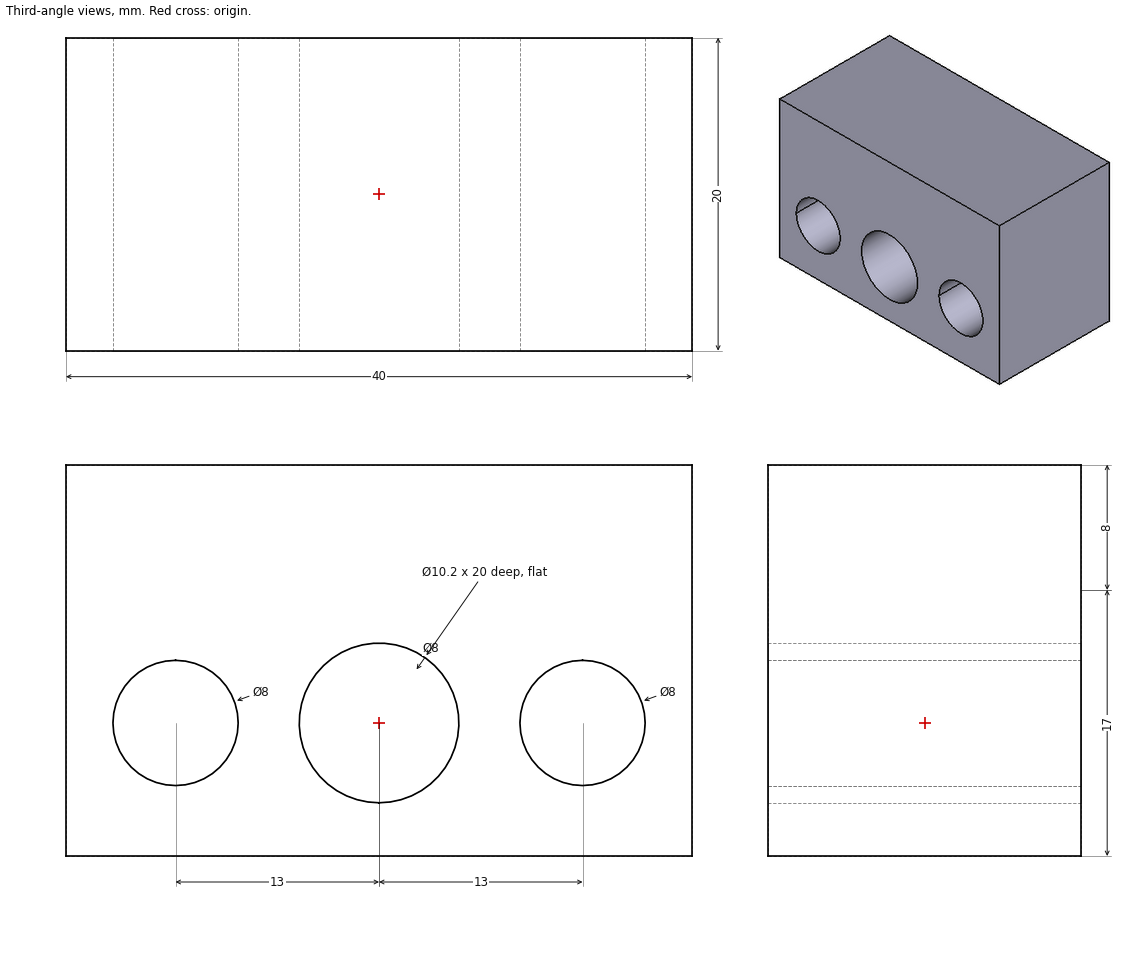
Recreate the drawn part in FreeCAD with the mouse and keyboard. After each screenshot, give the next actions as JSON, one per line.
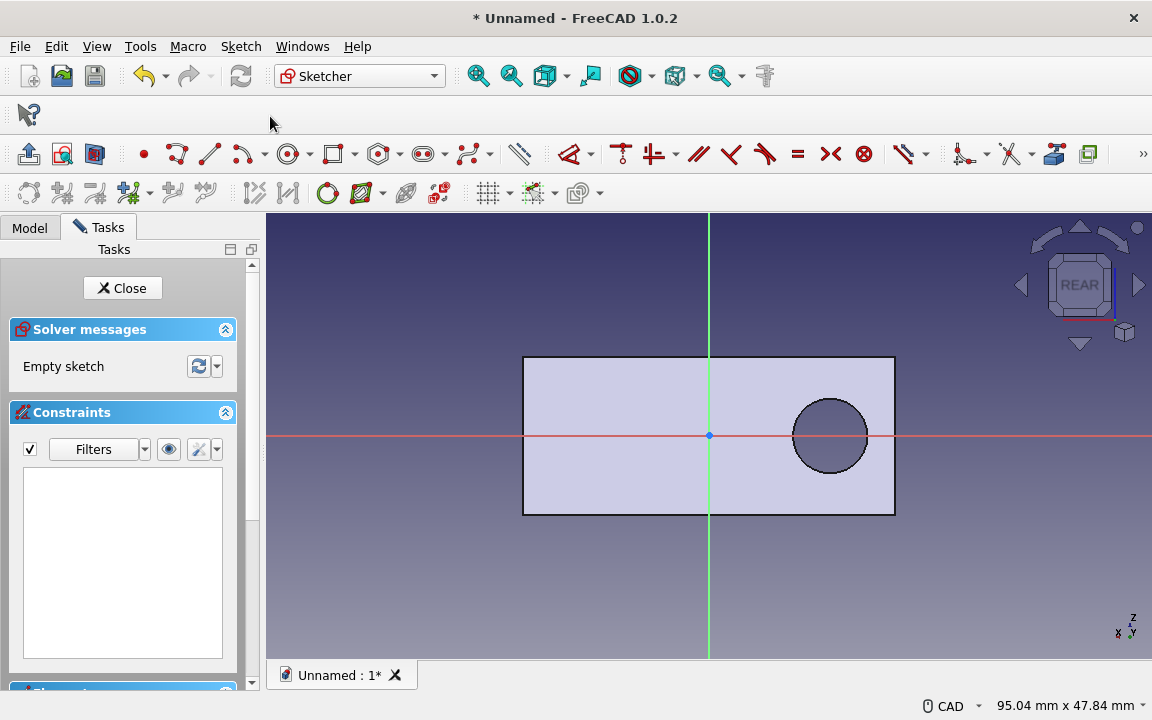
{"action": "scroll", "coordinate": [625, 436], "scroll_direction": "up", "scroll_amount": 6}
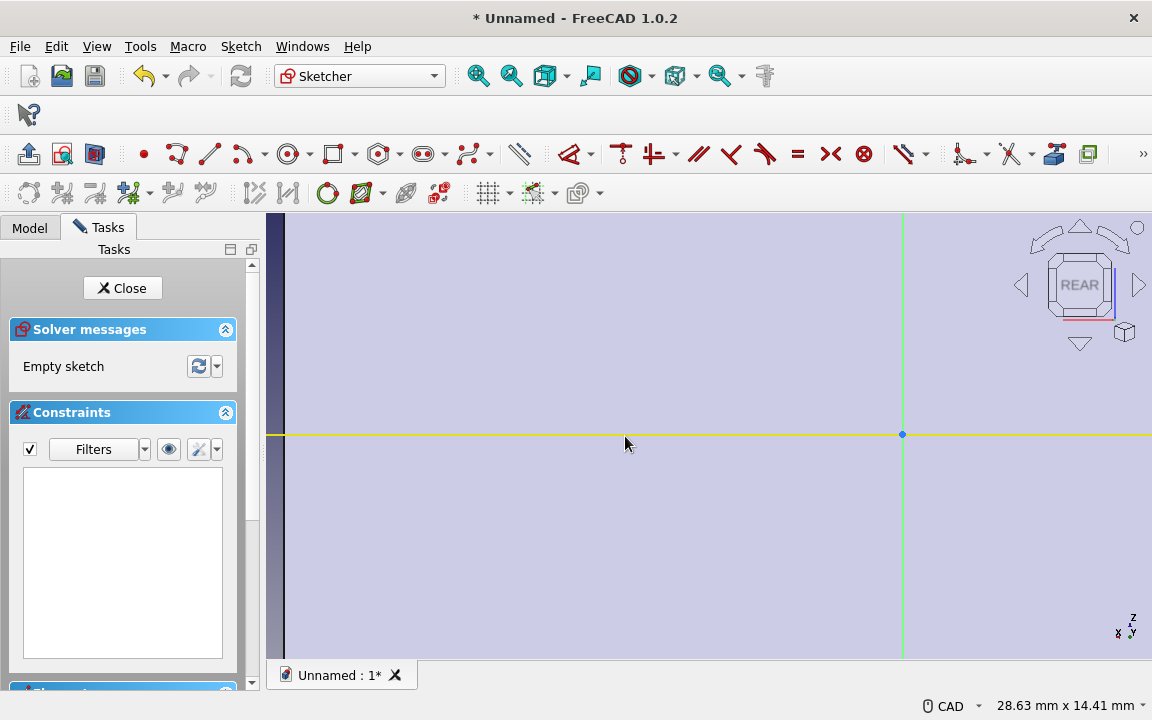
{"action": "left_click", "coordinate": [288, 154]}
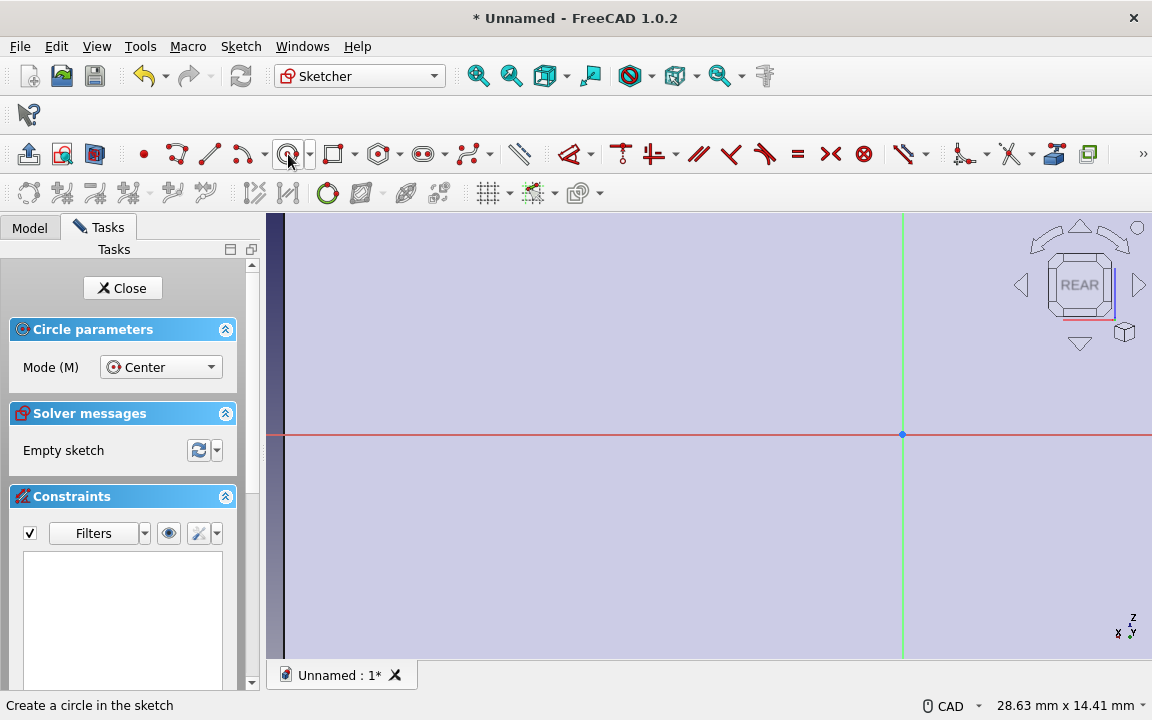
{"action": "left_click", "coordinate": [501, 435]}
{"action": "left_click", "coordinate": [588, 347]}
{"action": "key", "text": "Escape"}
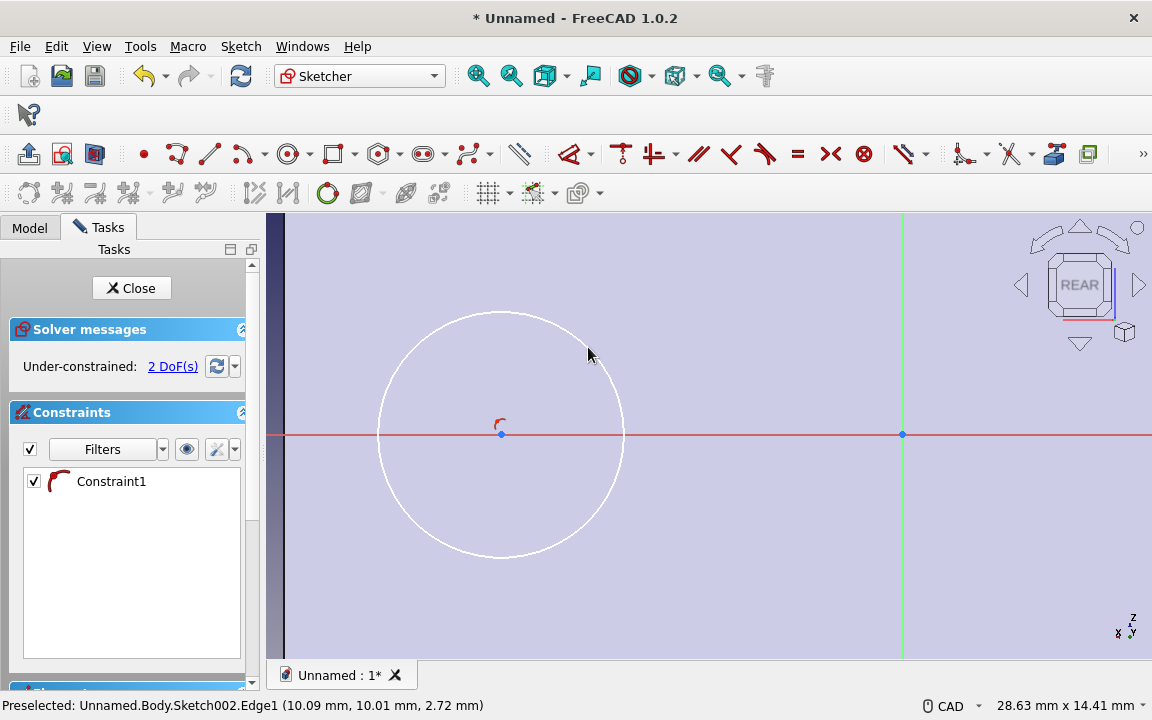
{"action": "left_click", "coordinate": [568, 154]}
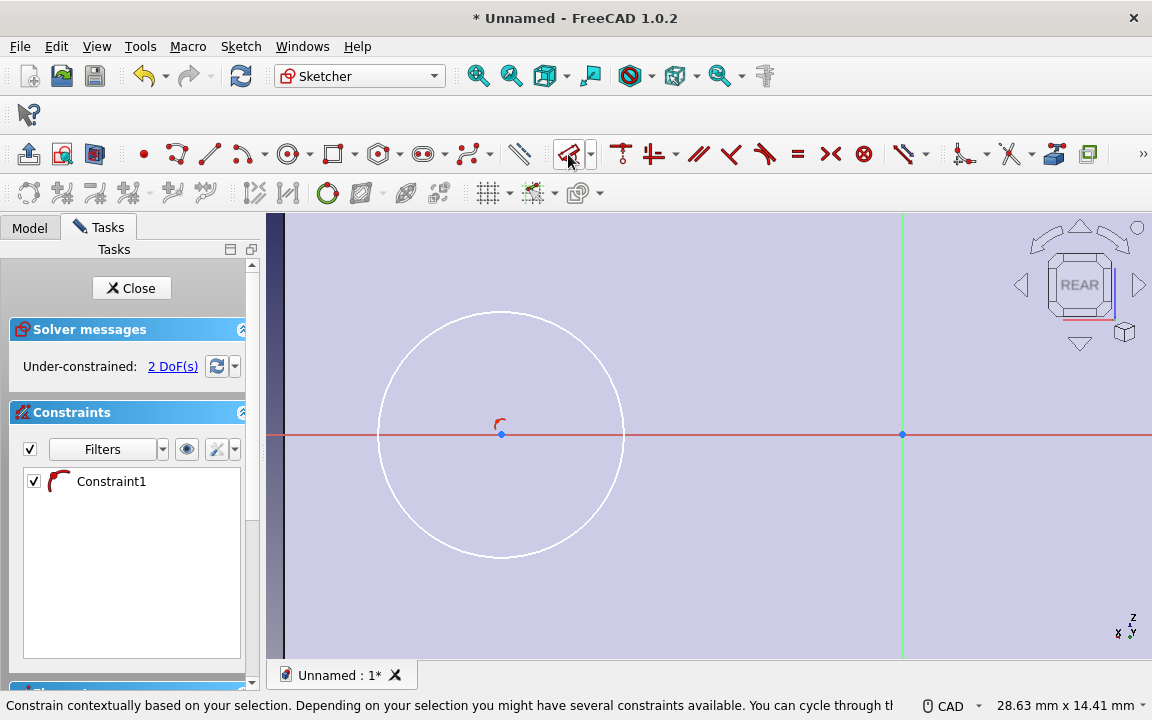
{"action": "left_click", "coordinate": [588, 348]}
{"action": "left_click", "coordinate": [611, 325]}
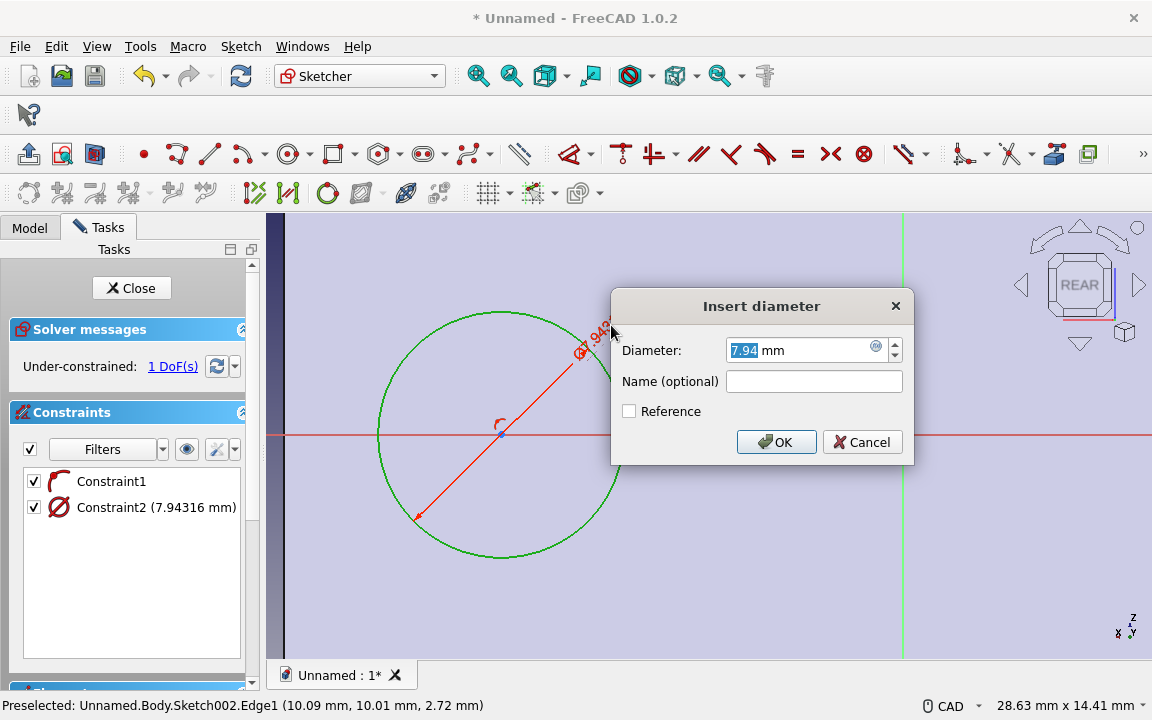
{"action": "type", "text": "8"}
{"action": "key", "text": "Return"}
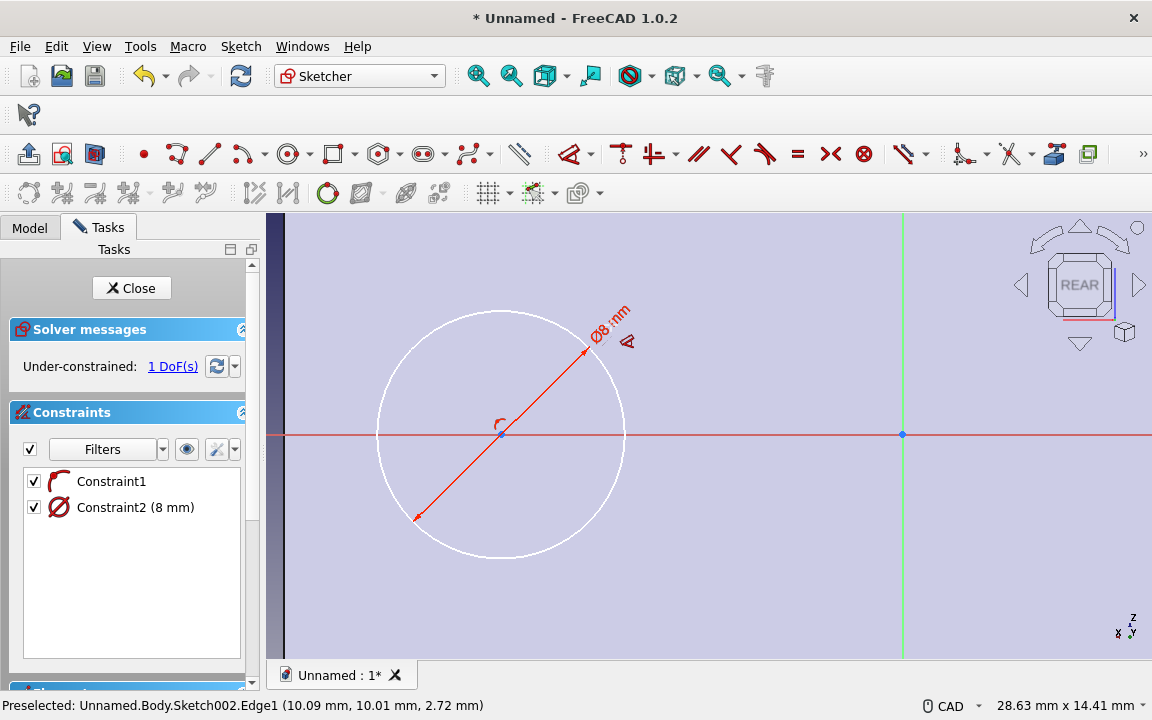
{"action": "left_click", "coordinate": [501, 435]}
{"action": "left_click", "coordinate": [702, 469]}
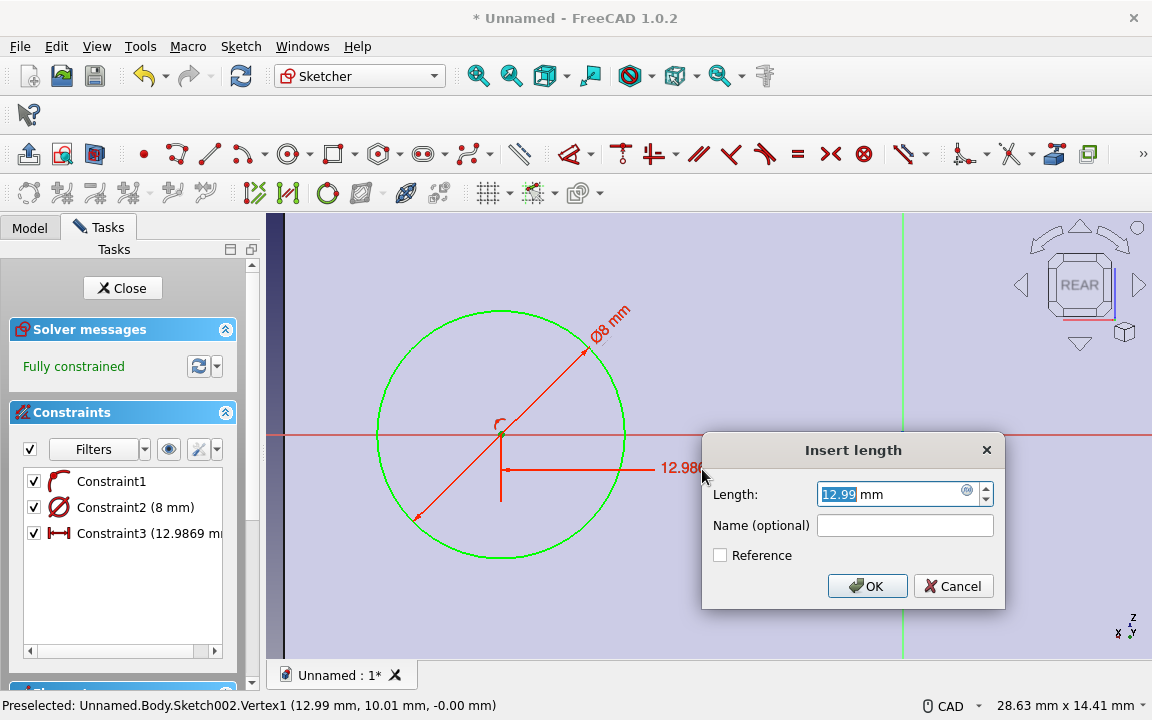
{"action": "type", "text": "13"}
{"action": "key", "text": "Return"}
{"action": "key", "text": "Escape"}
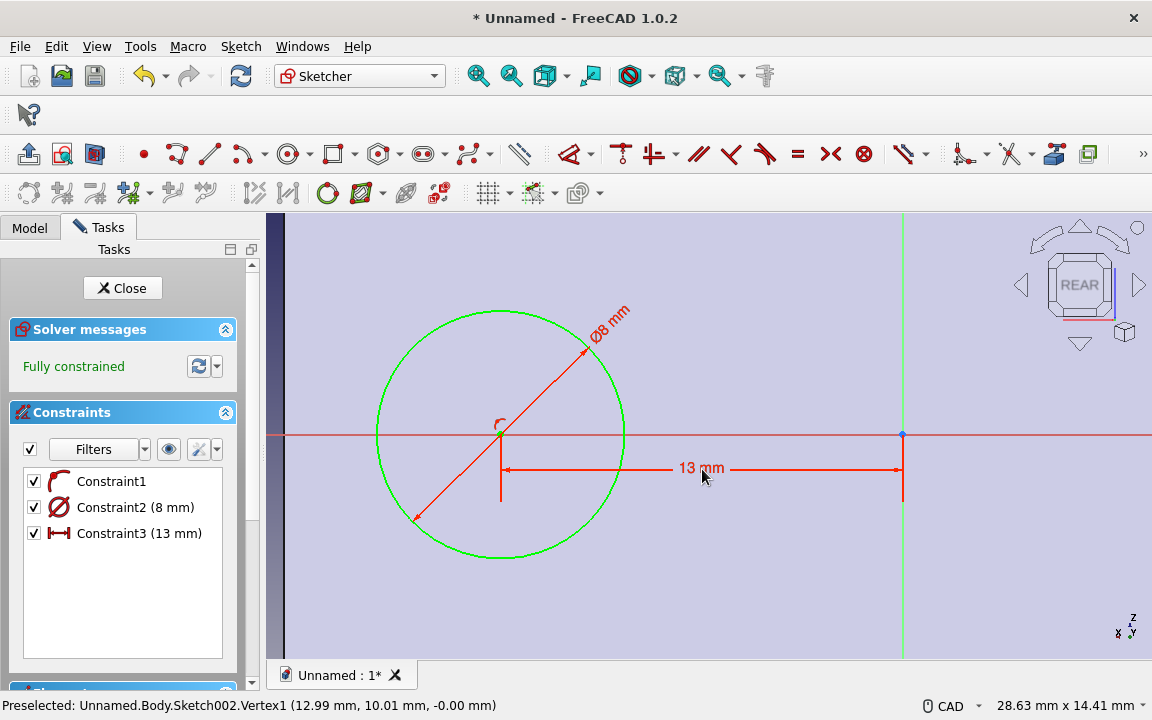
{"action": "left_click", "coordinate": [123, 288]}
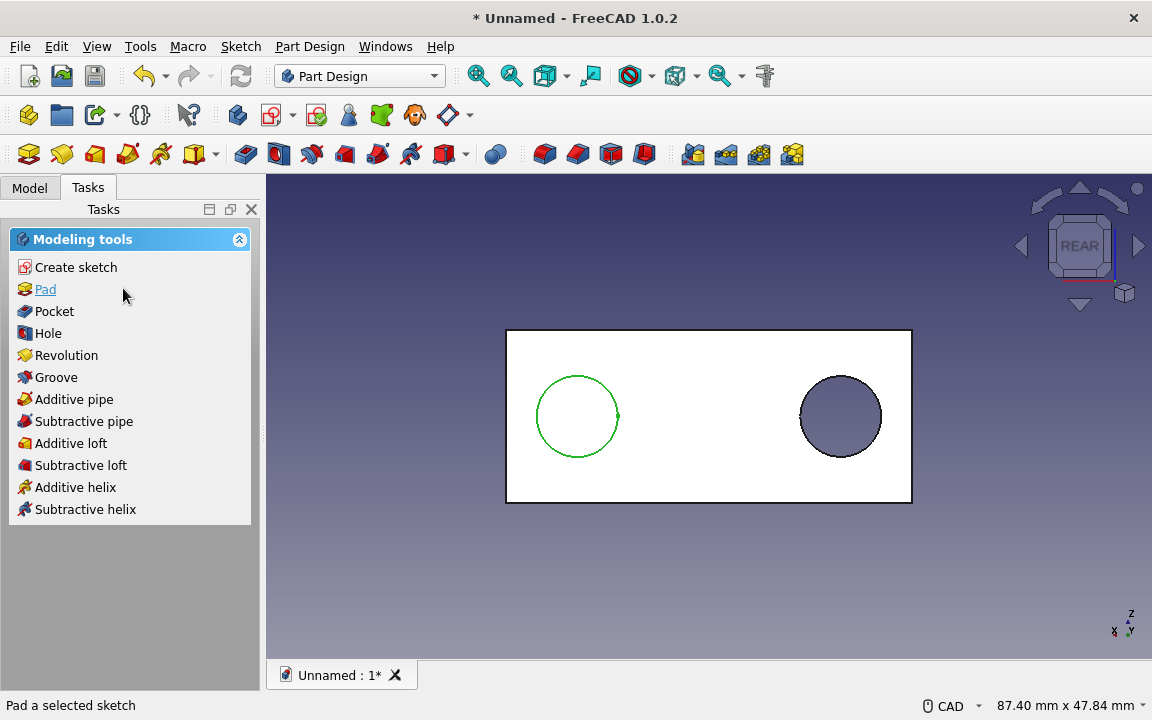
{"action": "left_click", "coordinate": [246, 154]}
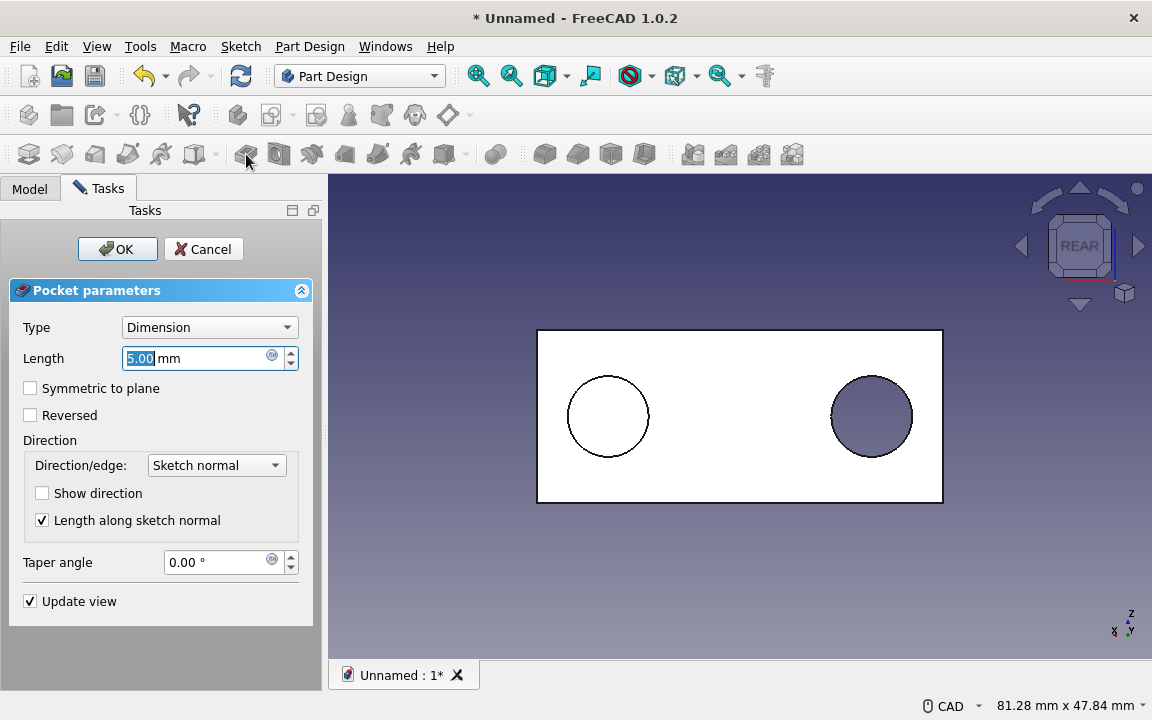
{"action": "left_click", "coordinate": [210, 328]}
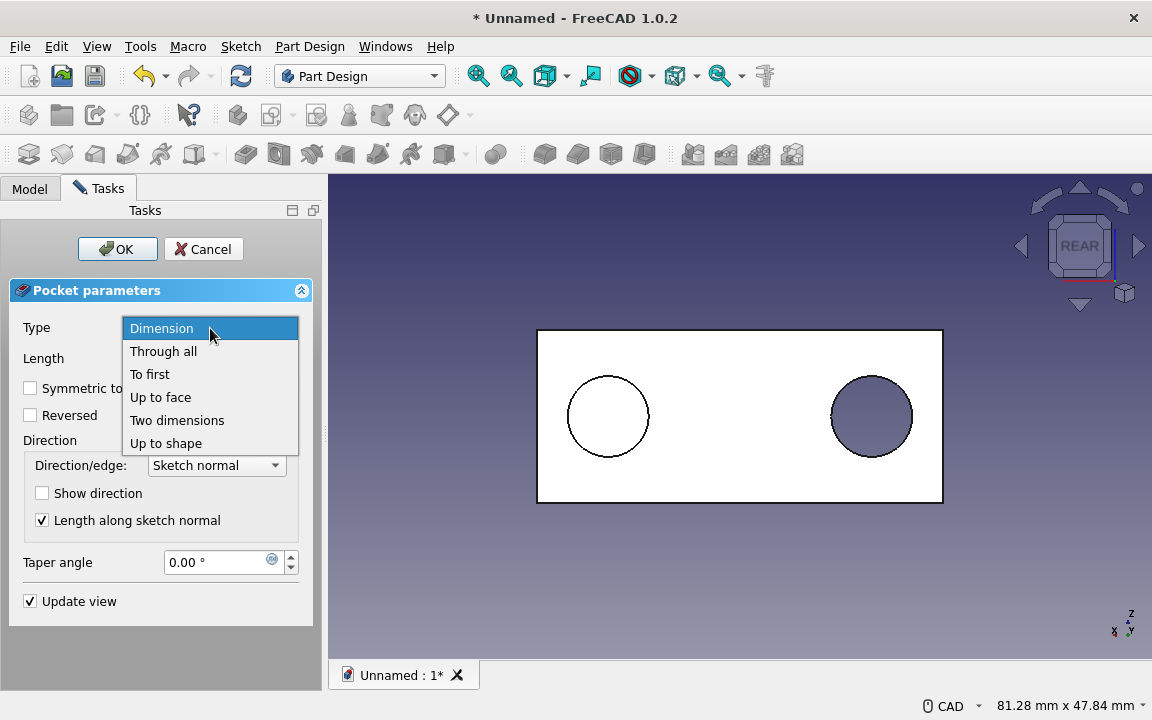
{"action": "left_click", "coordinate": [208, 374]}